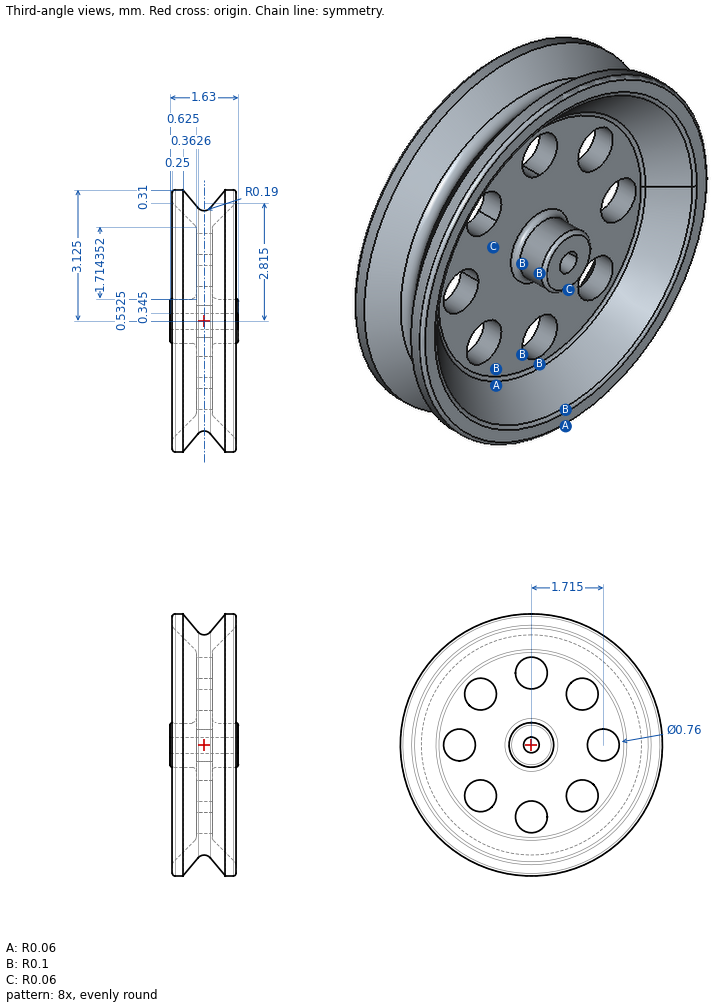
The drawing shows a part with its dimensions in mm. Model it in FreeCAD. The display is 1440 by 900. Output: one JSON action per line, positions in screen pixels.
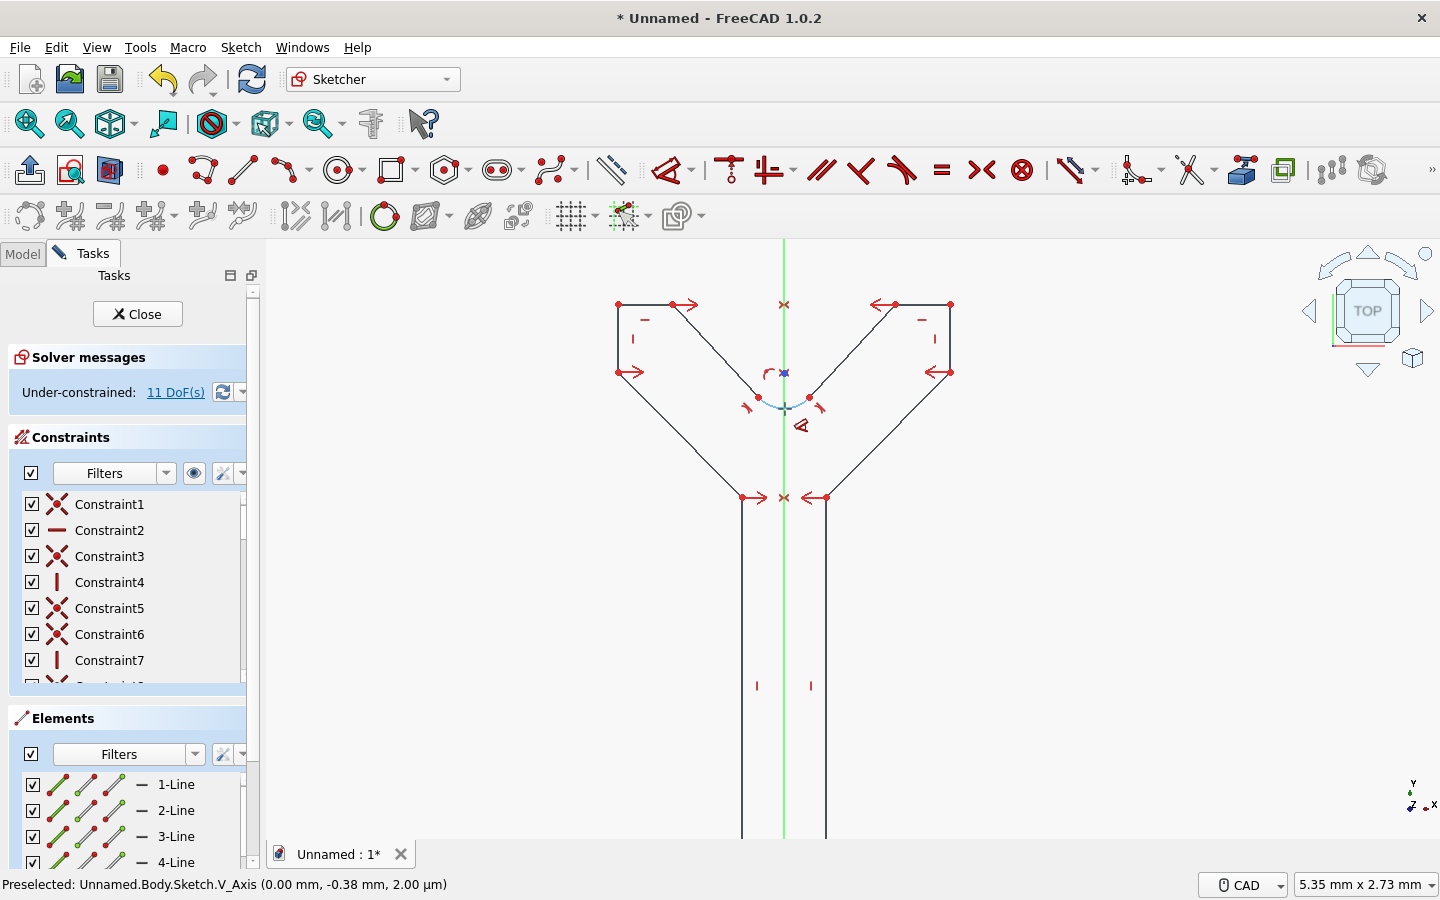
{"action": "left_click", "coordinate": [784, 408]}
{"action": "left_click", "coordinate": [752, 432]}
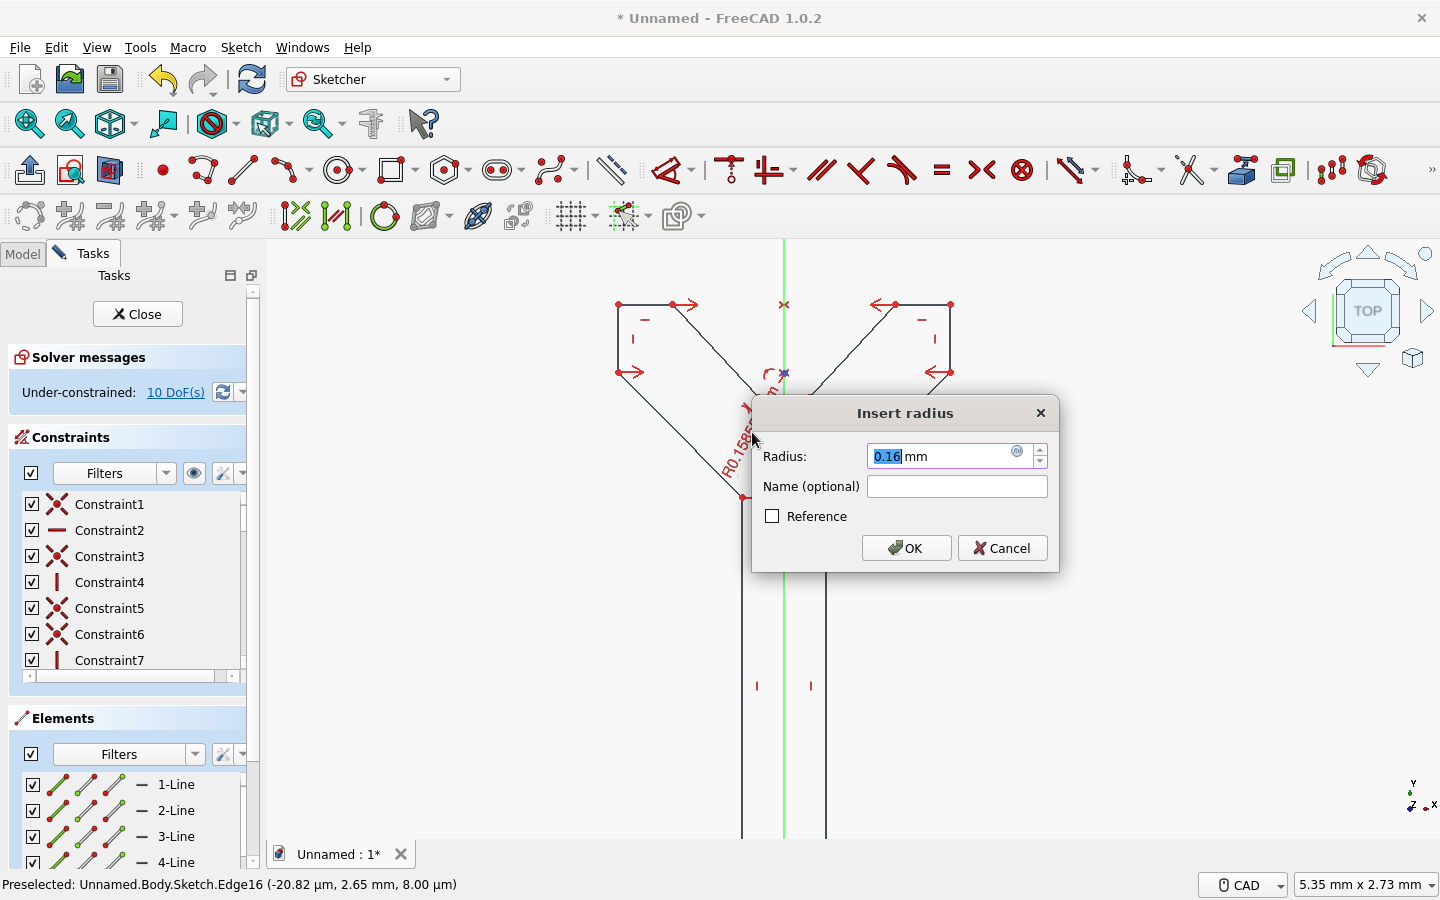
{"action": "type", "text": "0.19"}
{"action": "key", "text": "Return"}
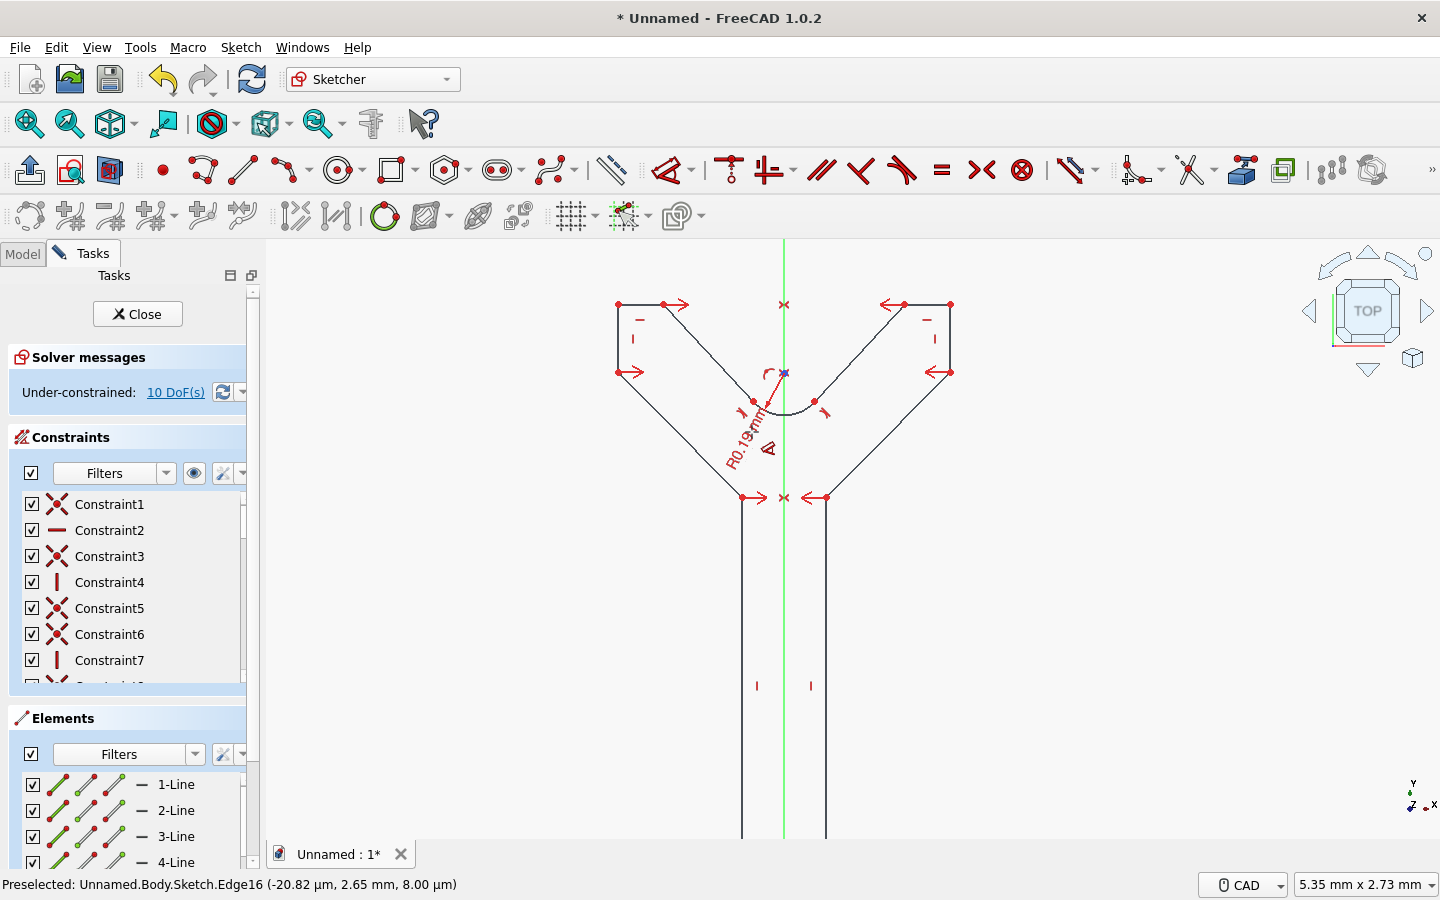
{"action": "left_click", "coordinate": [650, 305]}
{"action": "left_click", "coordinate": [641, 271]}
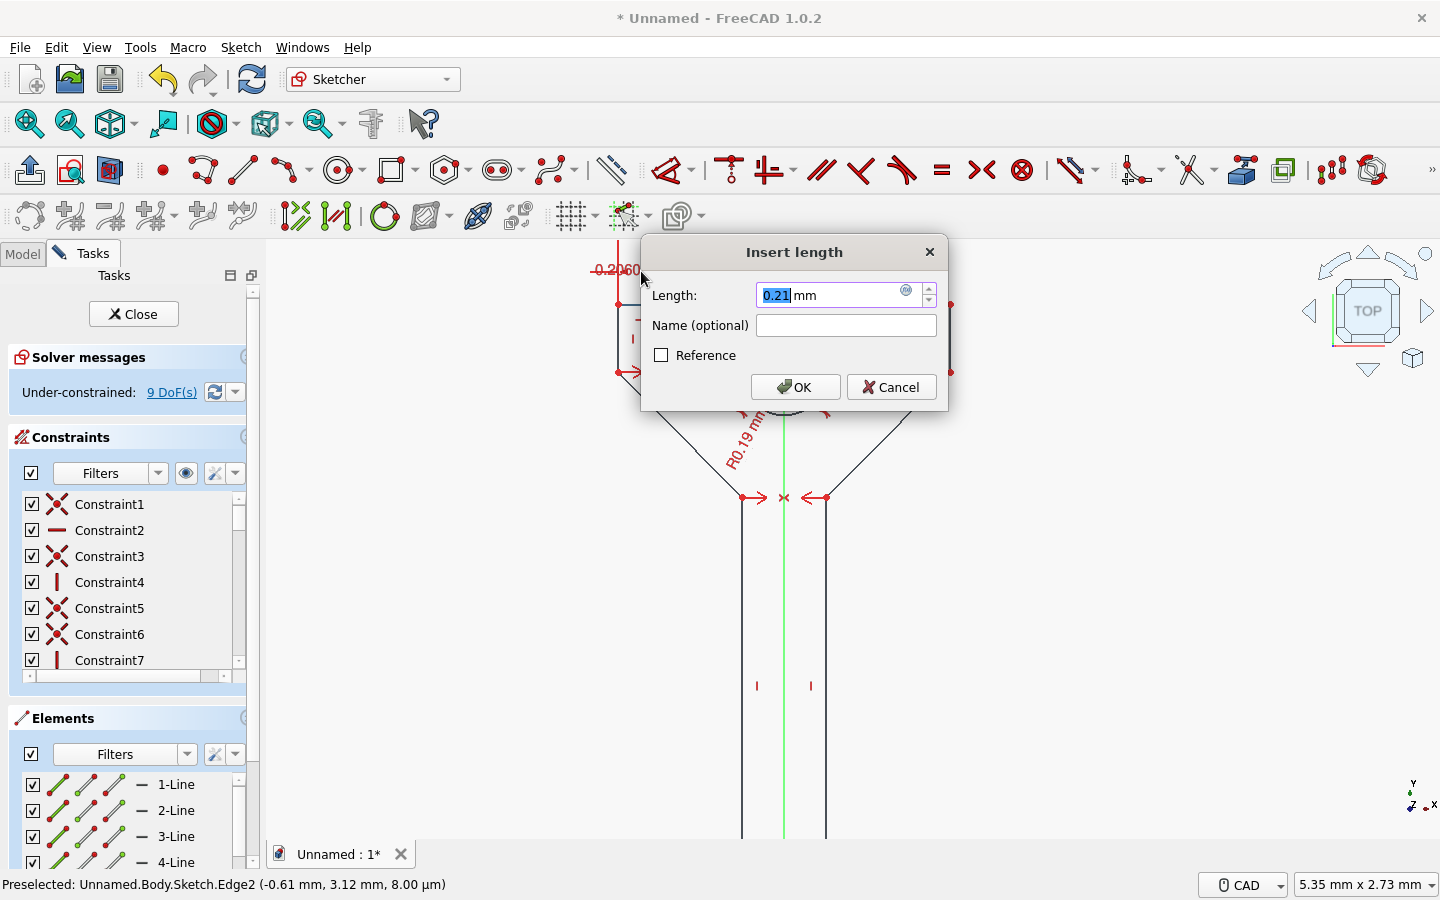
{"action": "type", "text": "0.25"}
{"action": "key", "text": "Return"}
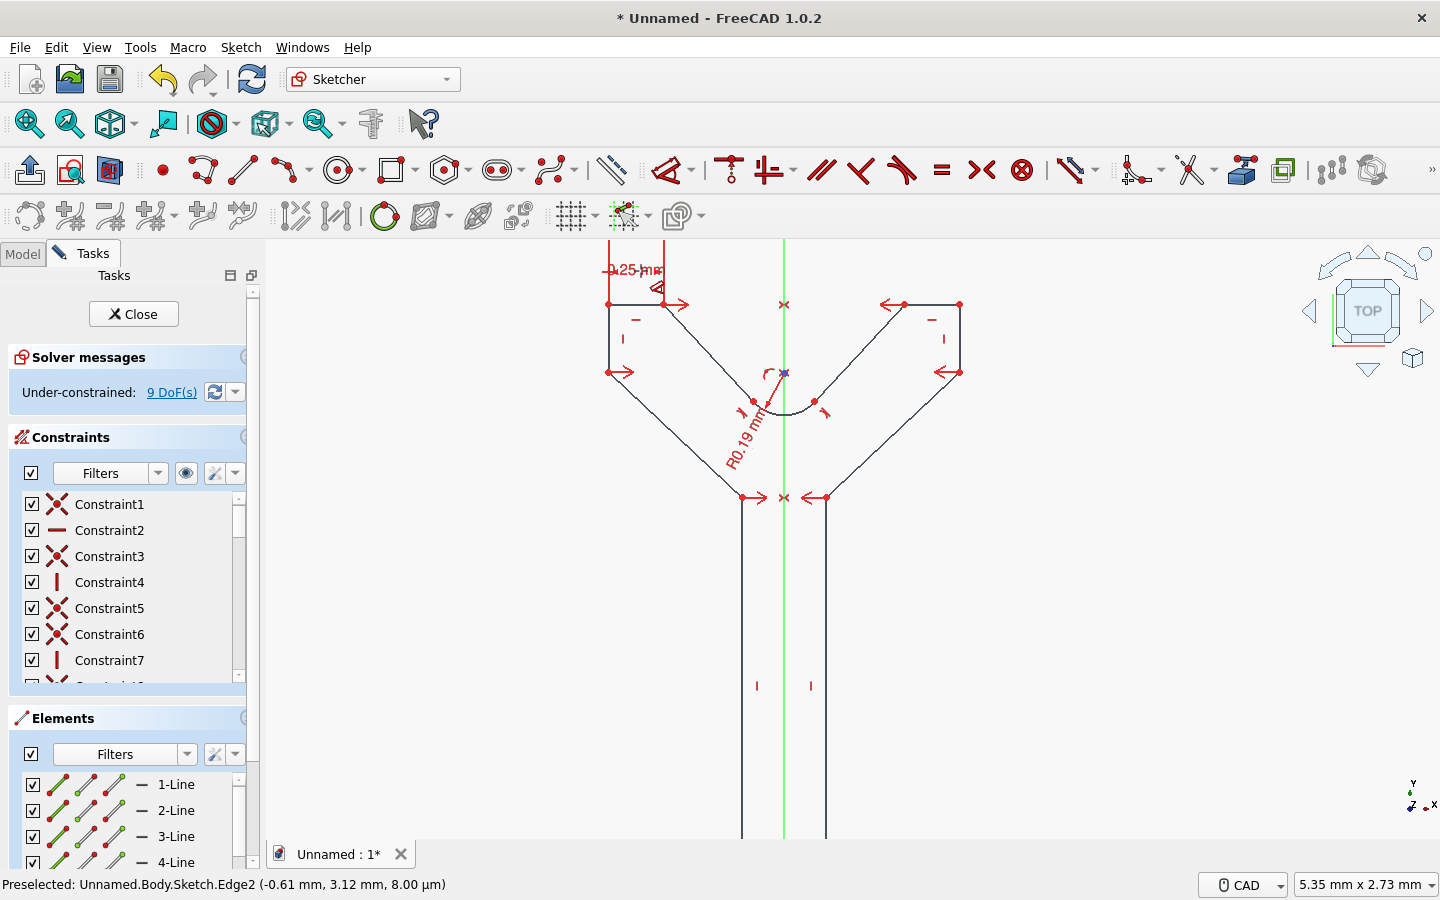
{"action": "left_click", "coordinate": [609, 325]}
{"action": "left_click", "coordinate": [575, 339]}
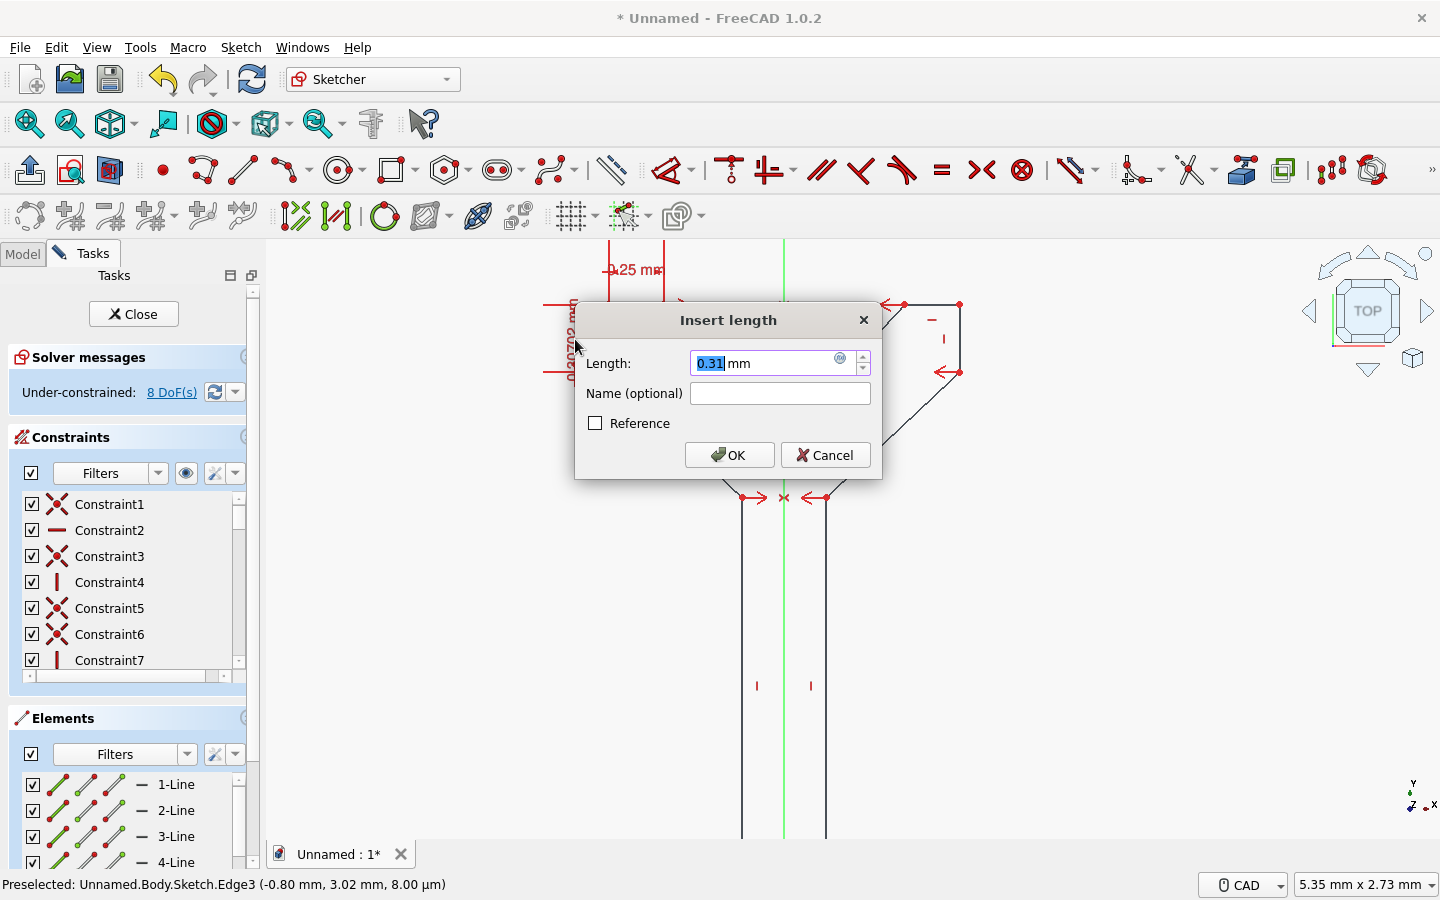
{"action": "type", "text": "0.31"}
{"action": "key", "text": "Return"}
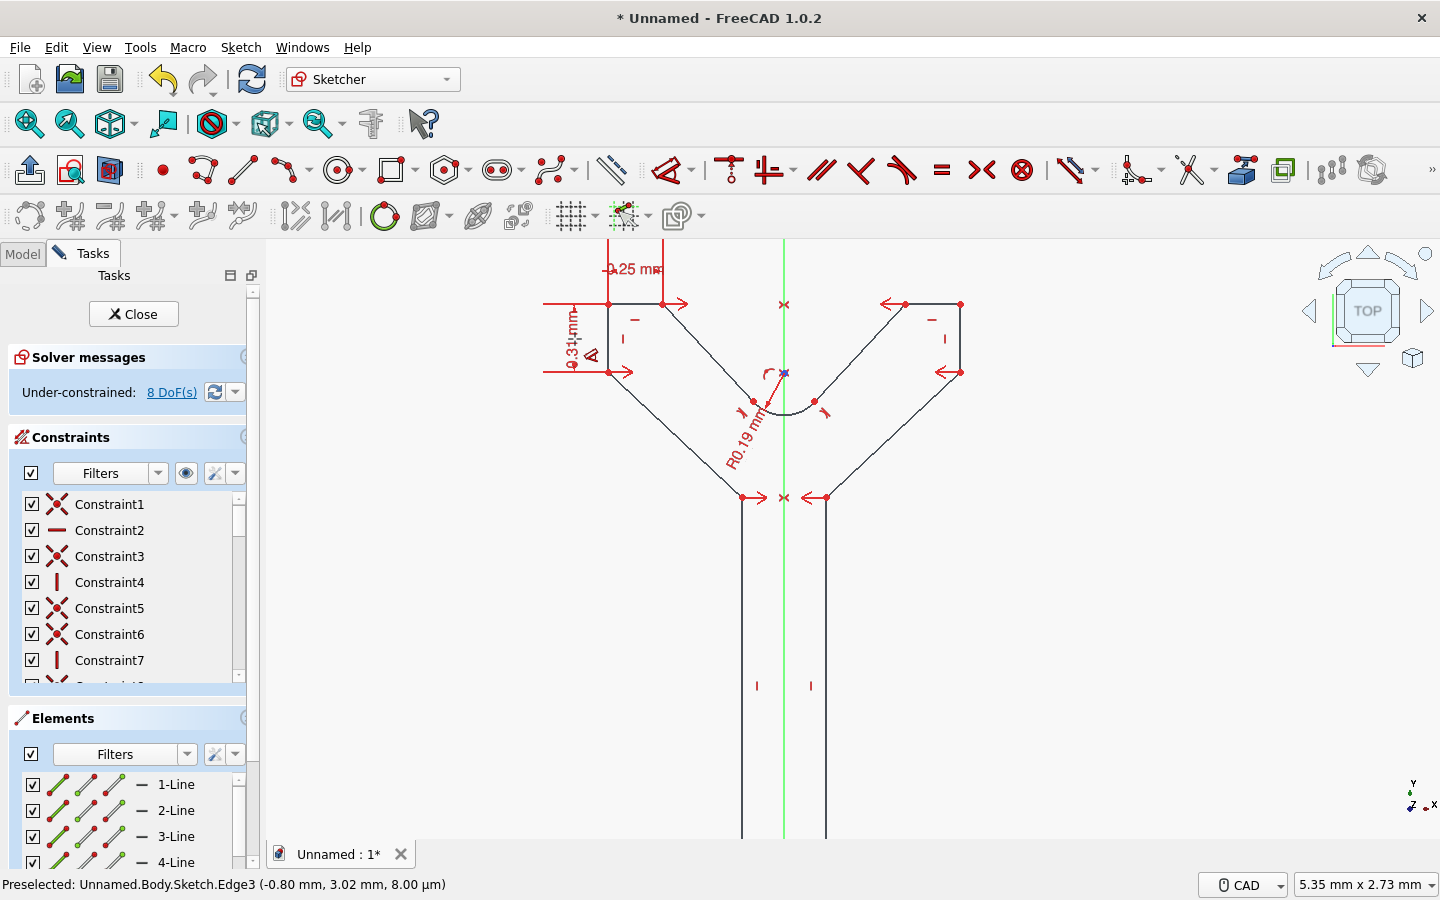
{"action": "scroll", "coordinate": [785, 409], "scroll_direction": "down", "scroll_amount": 3}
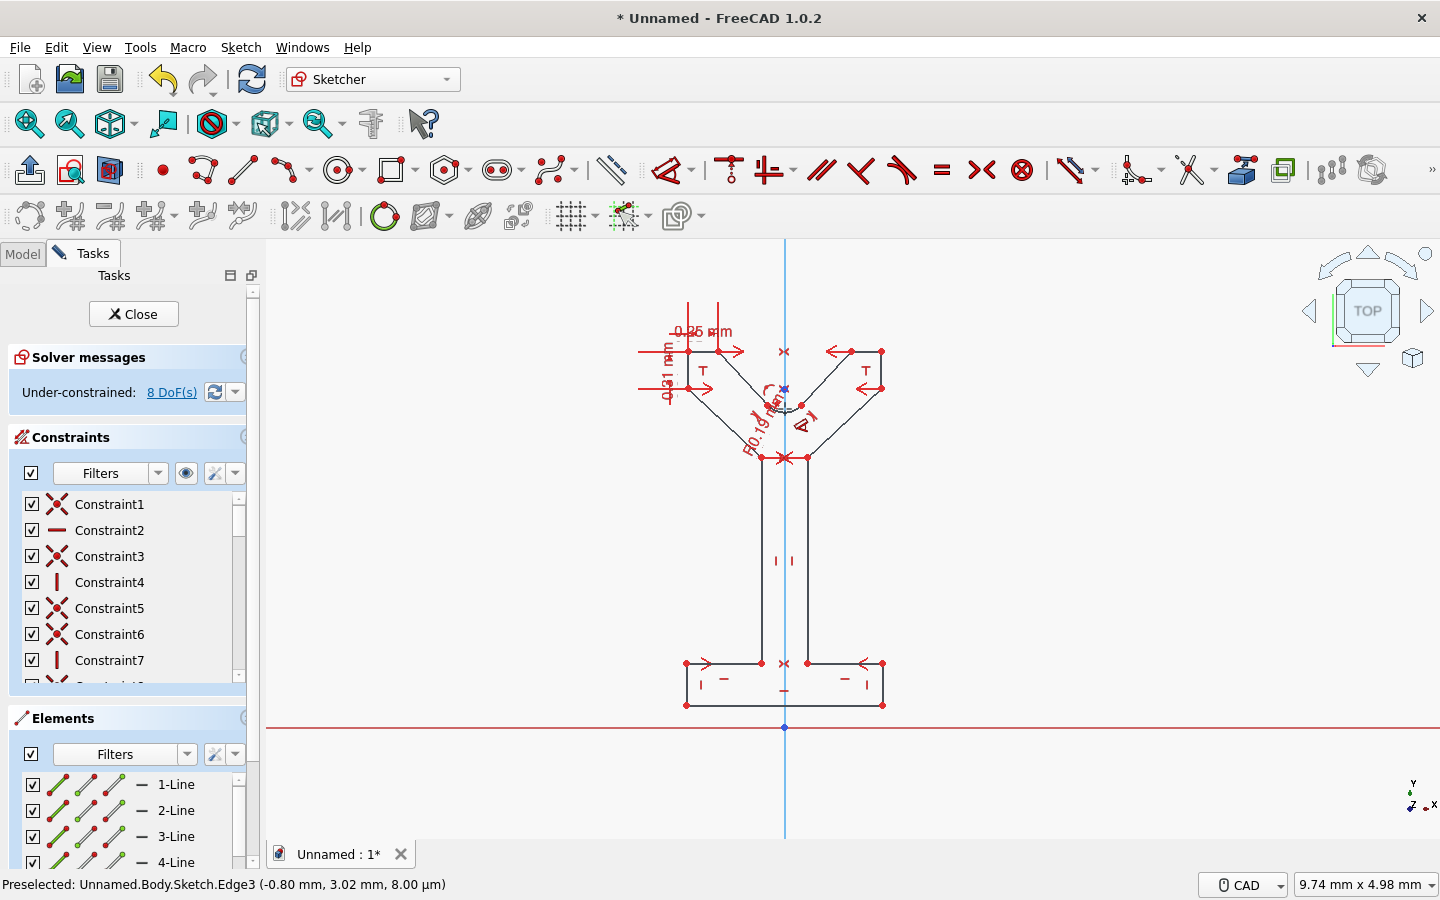
{"action": "left_click", "coordinate": [746, 706]}
{"action": "left_click", "coordinate": [740, 764]}